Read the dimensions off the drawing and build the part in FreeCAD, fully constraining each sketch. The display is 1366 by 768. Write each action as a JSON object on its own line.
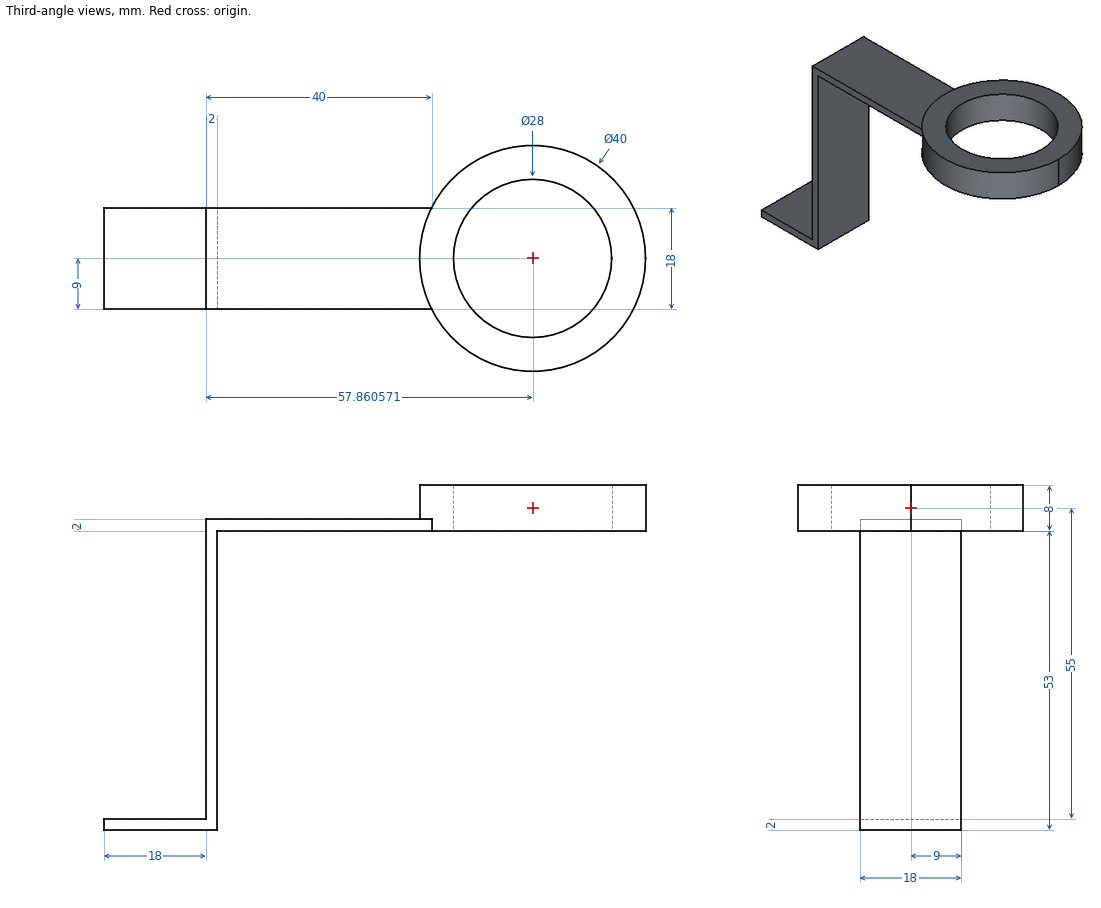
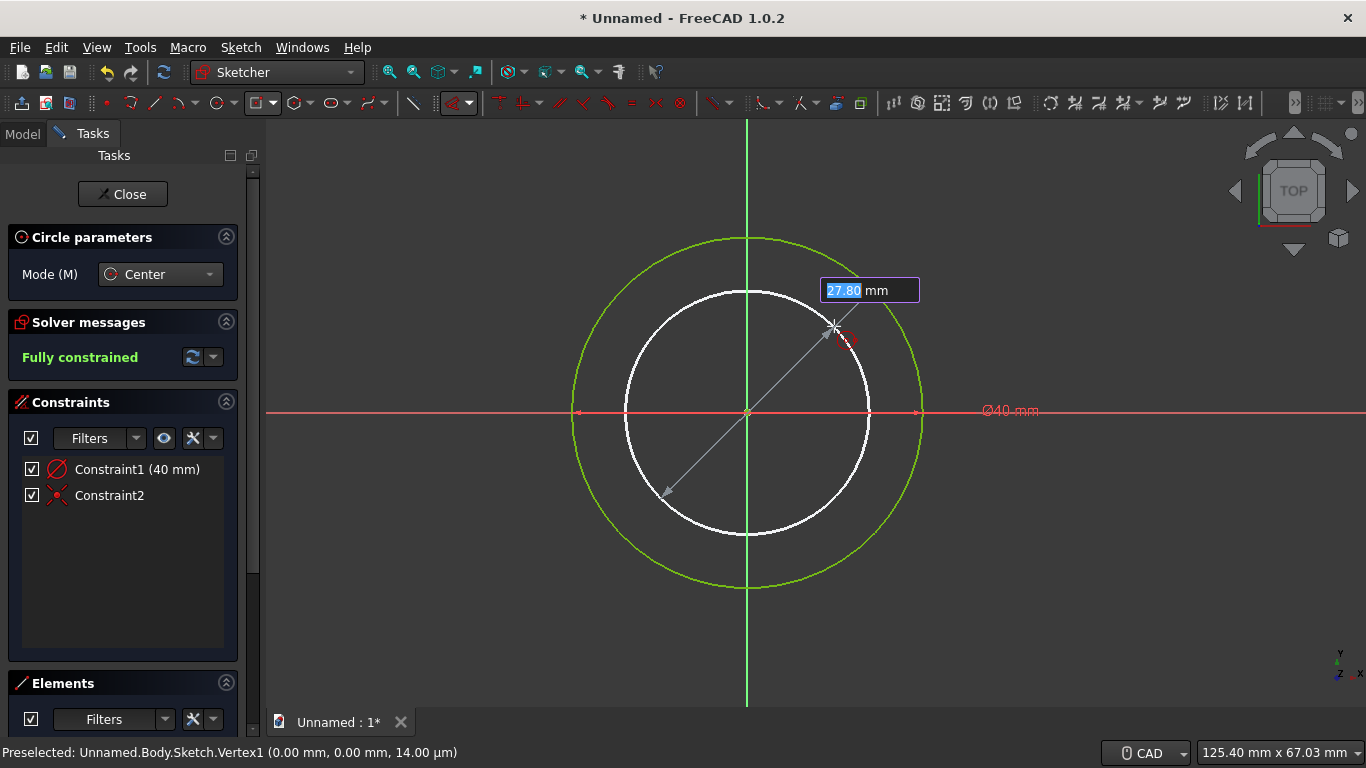
{"action": "type", "text": "28"}
{"action": "key", "text": "Return"}
{"action": "key", "text": "Escape"}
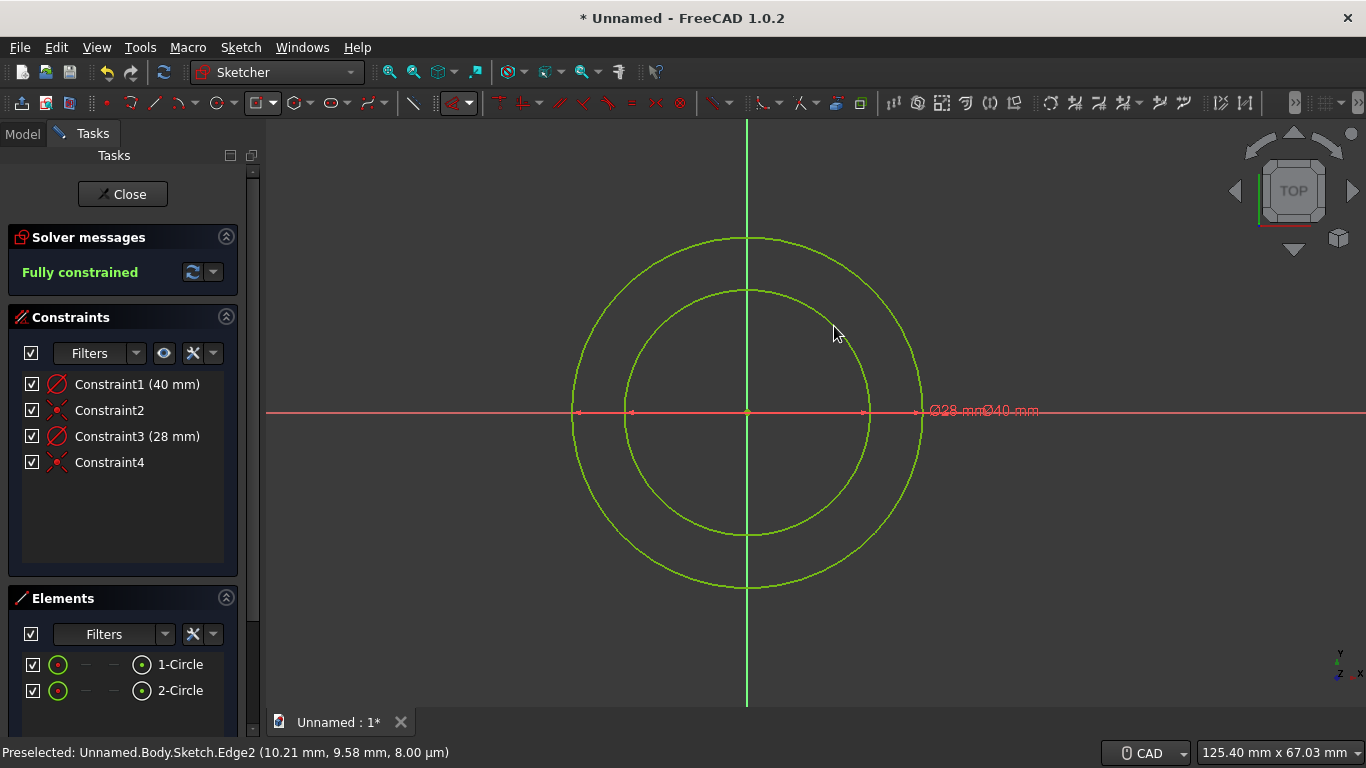
{"action": "left_click", "coordinate": [123, 194]}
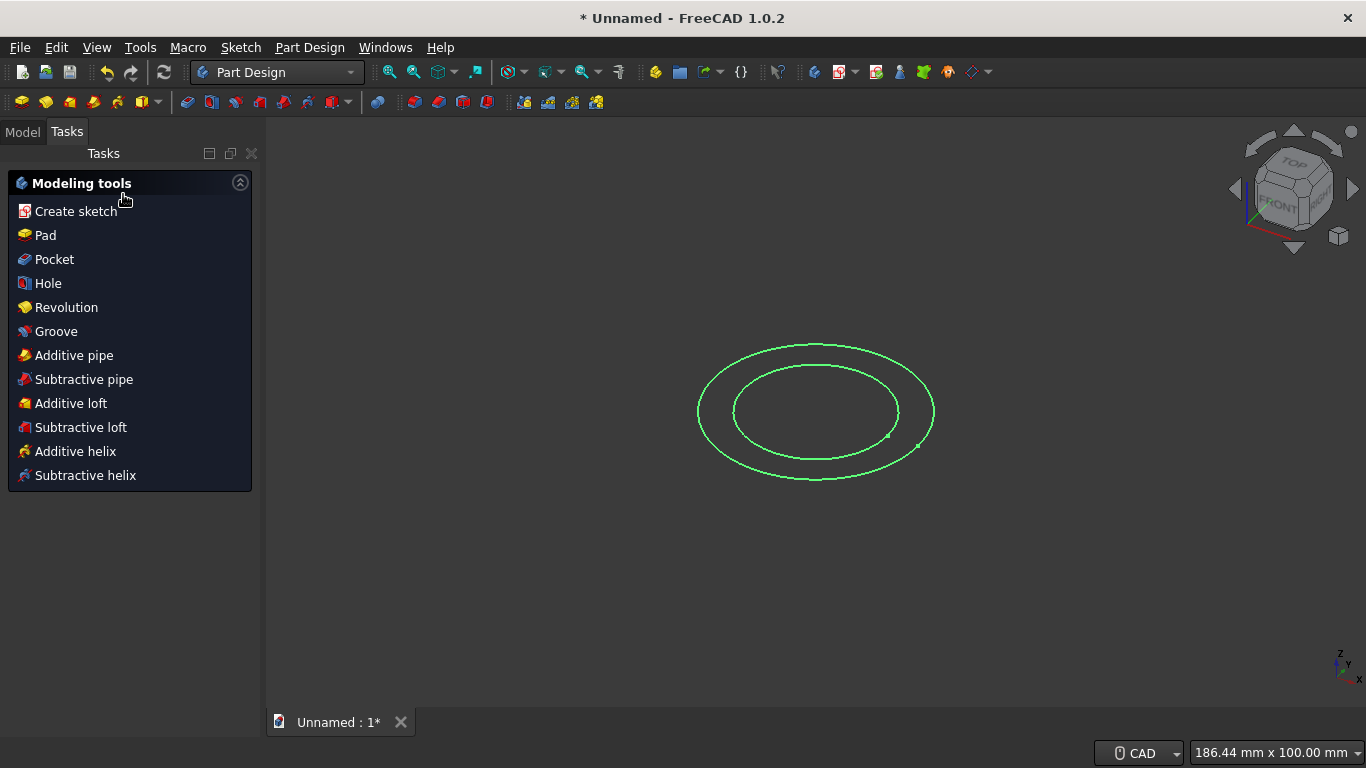
{"action": "left_click", "coordinate": [22, 102]}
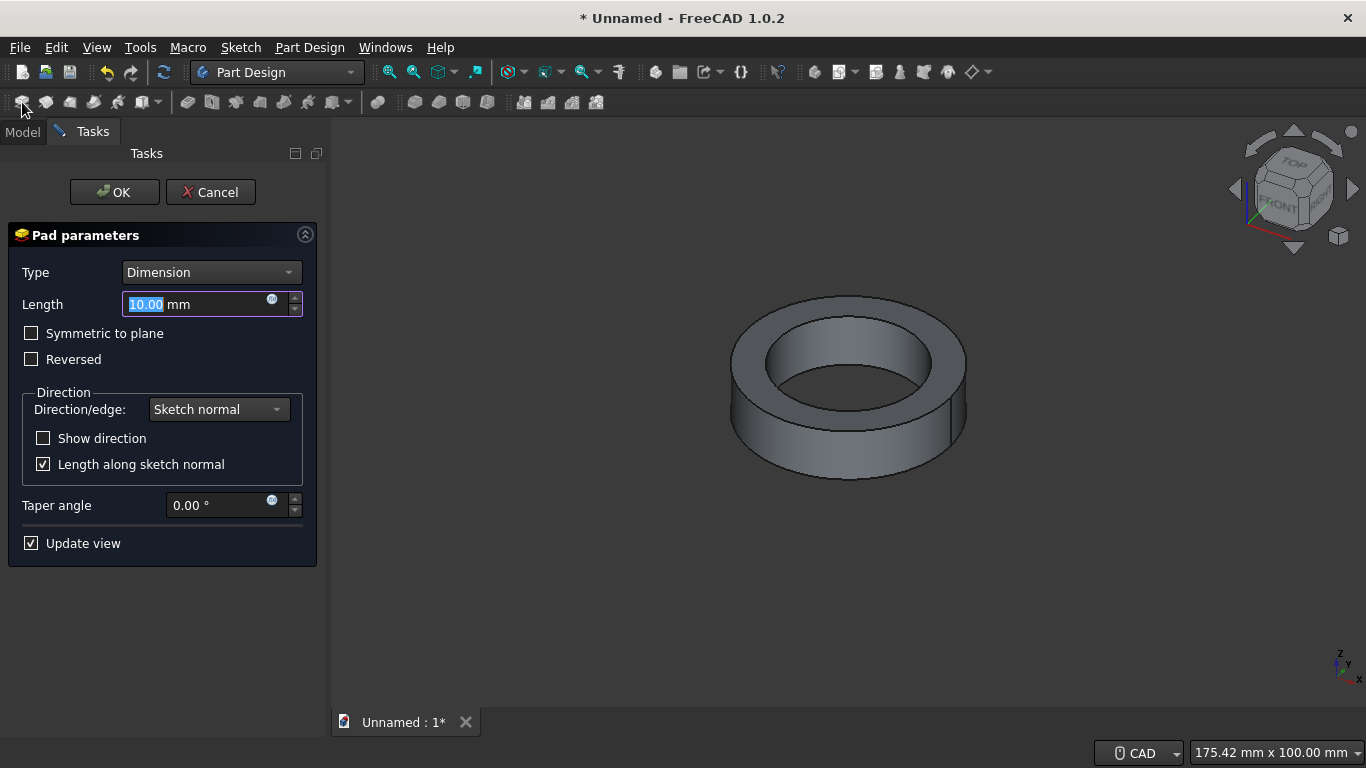
{"action": "type", "text": "8"}
{"action": "key", "text": "Tab"}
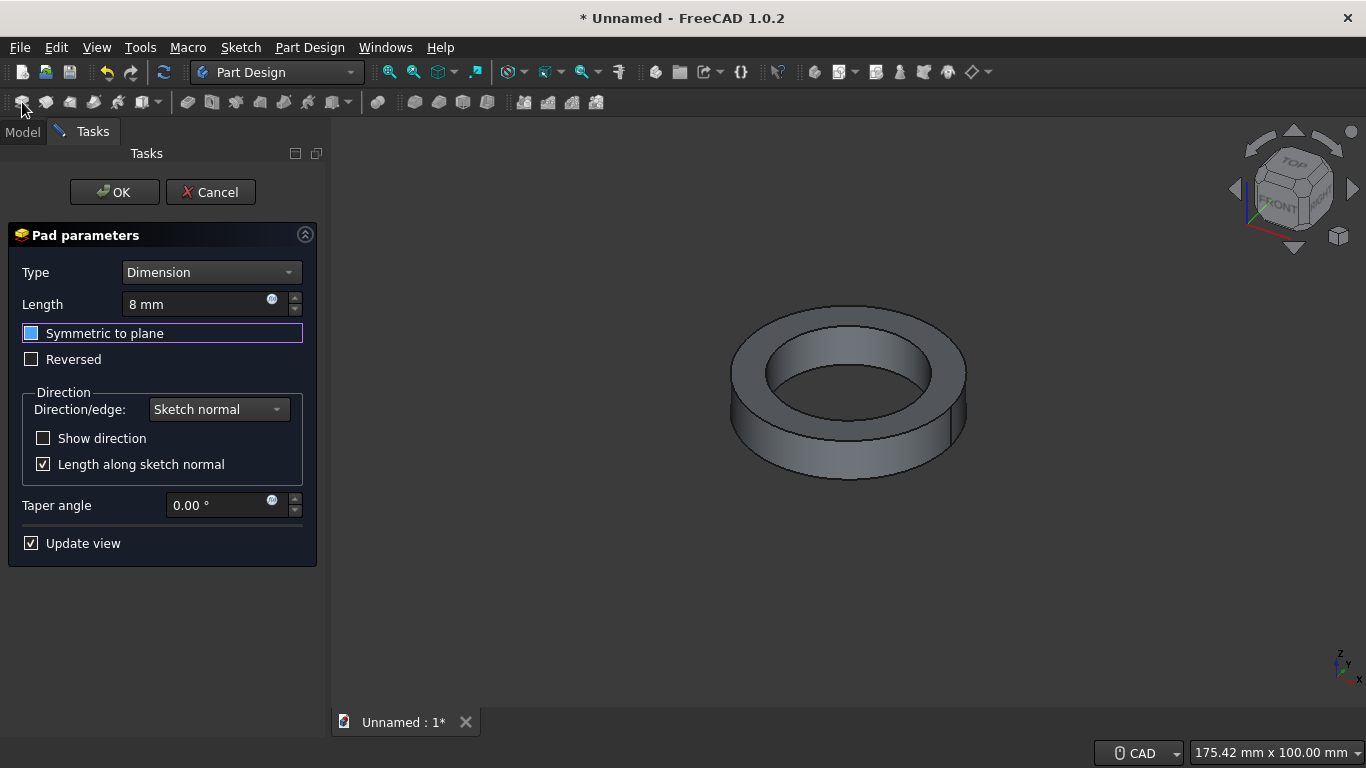
{"action": "left_click", "coordinate": [30, 333]}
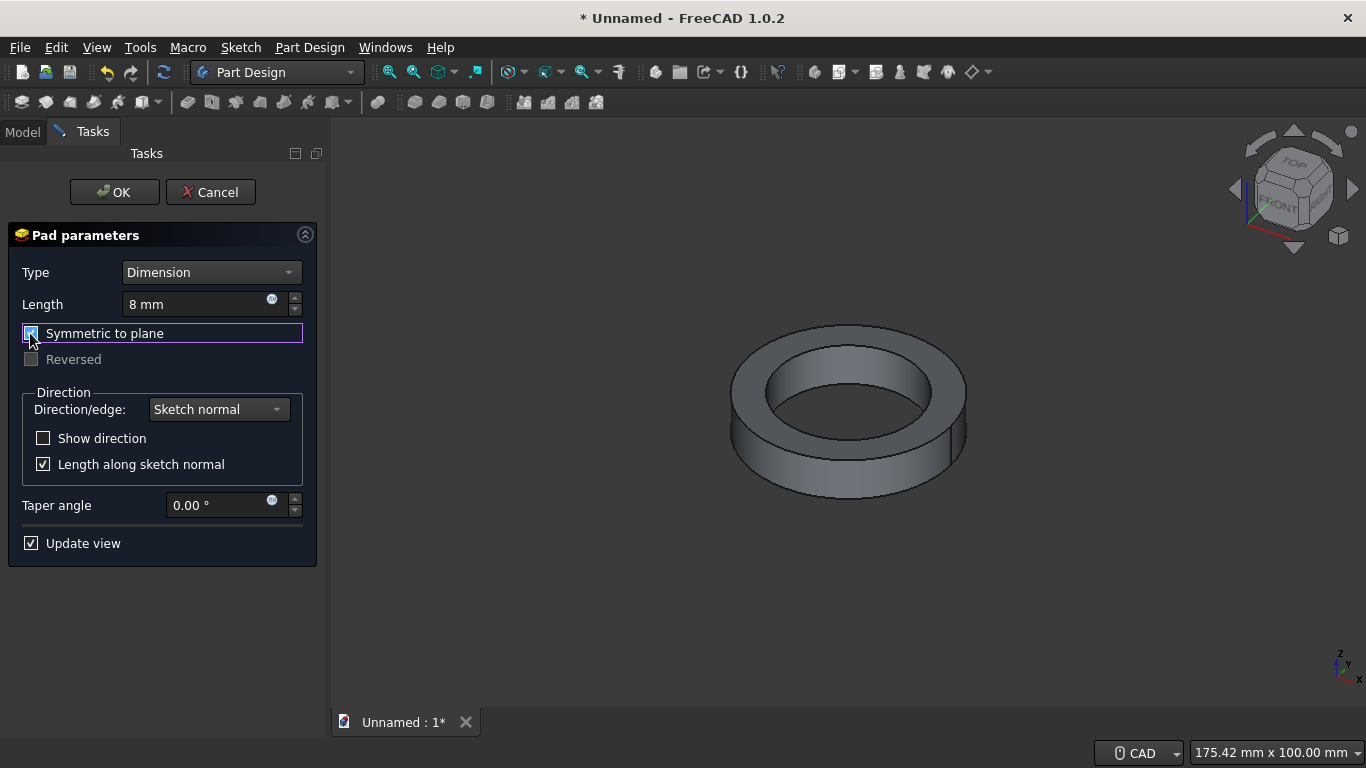
{"action": "left_click", "coordinate": [115, 192]}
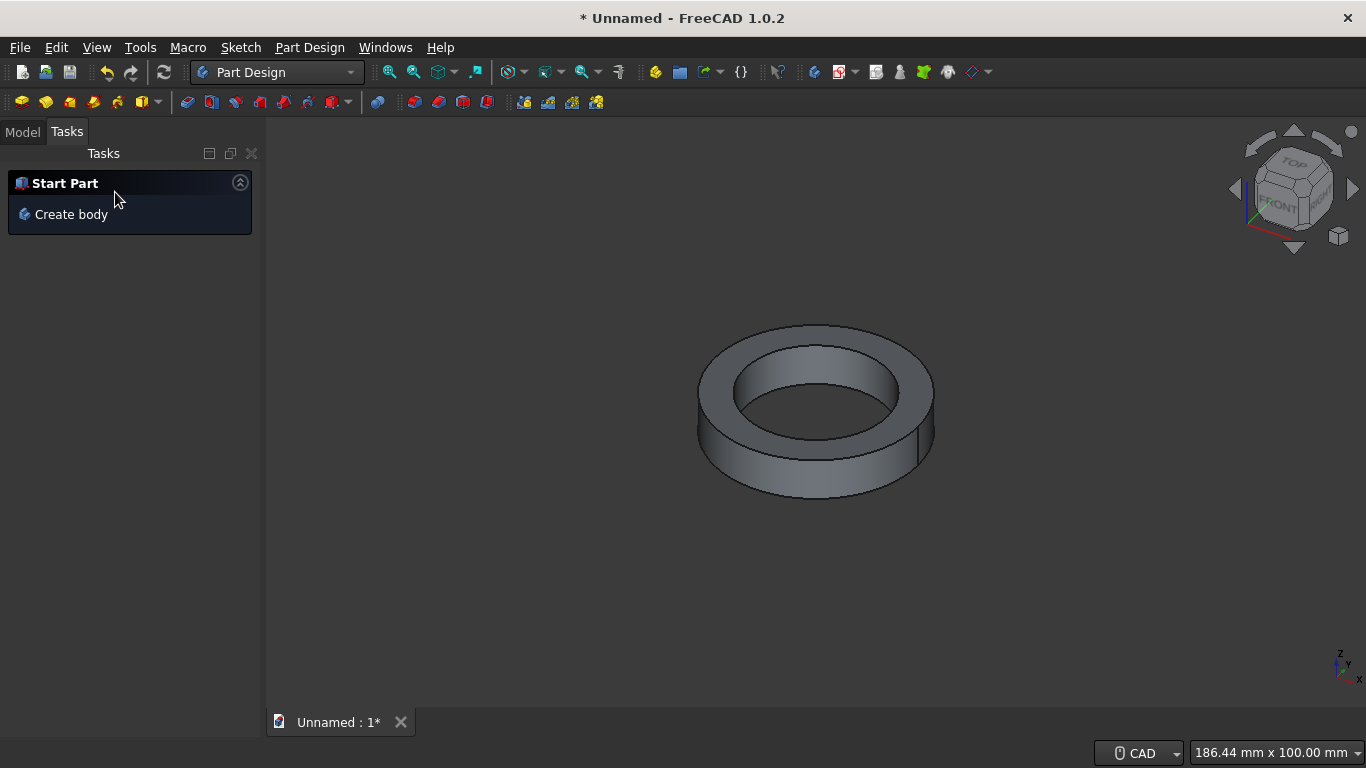
{"action": "left_click", "coordinate": [390, 72]}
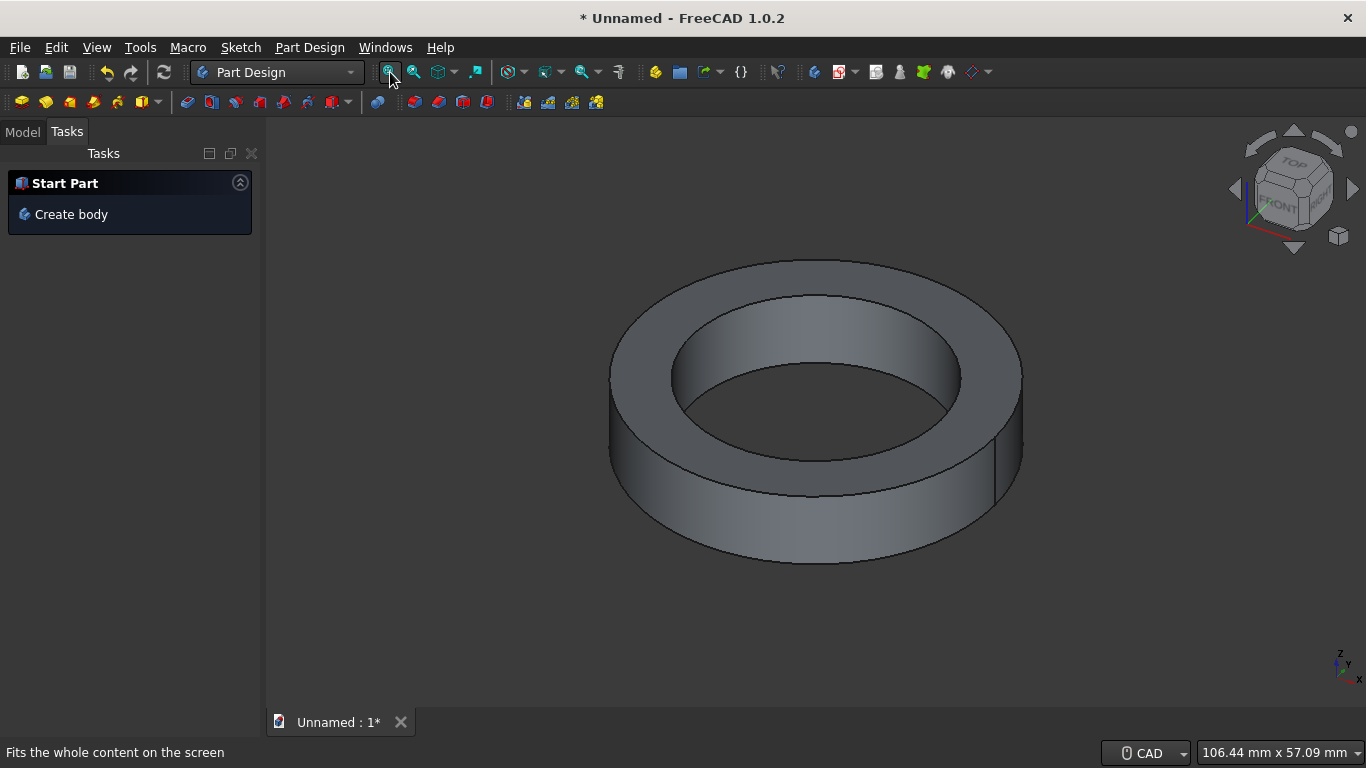
{"action": "key", "text": "5"}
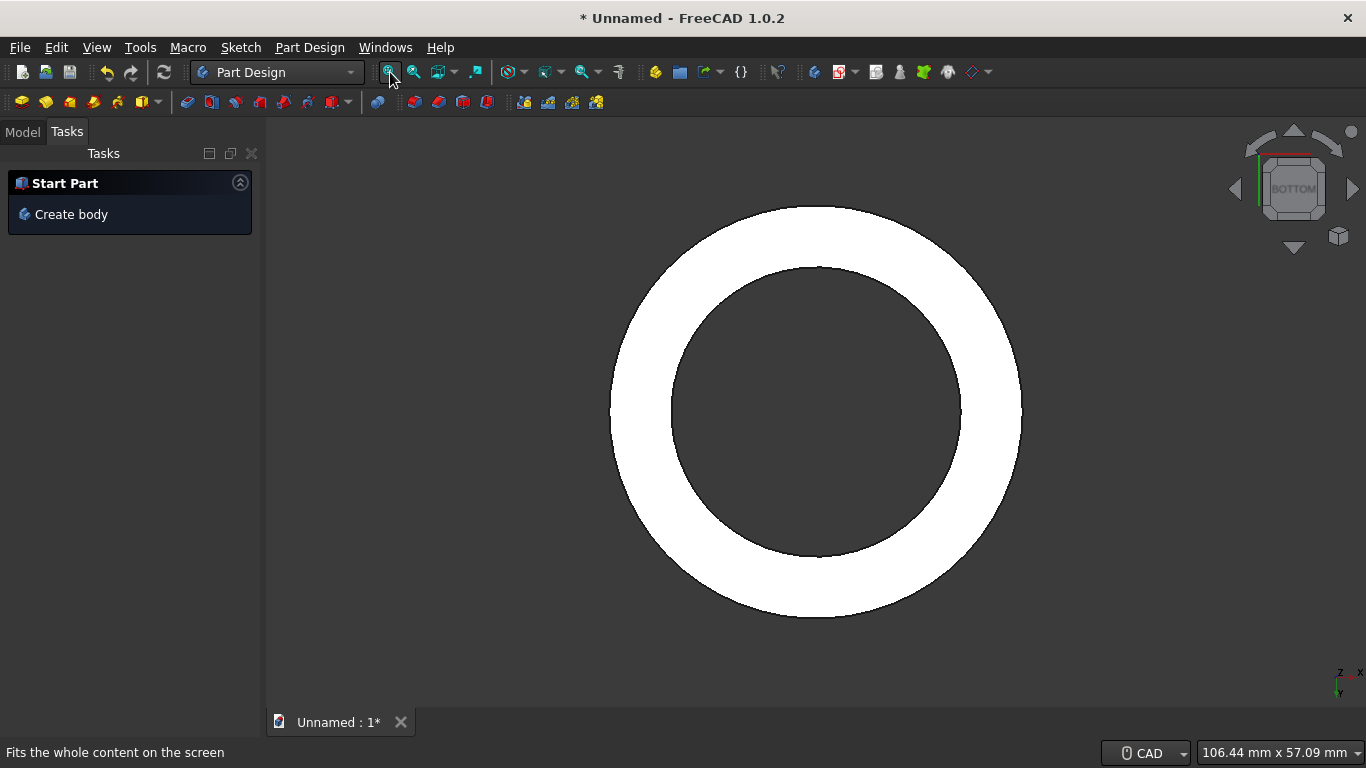
{"action": "left_click", "coordinate": [816, 234]}